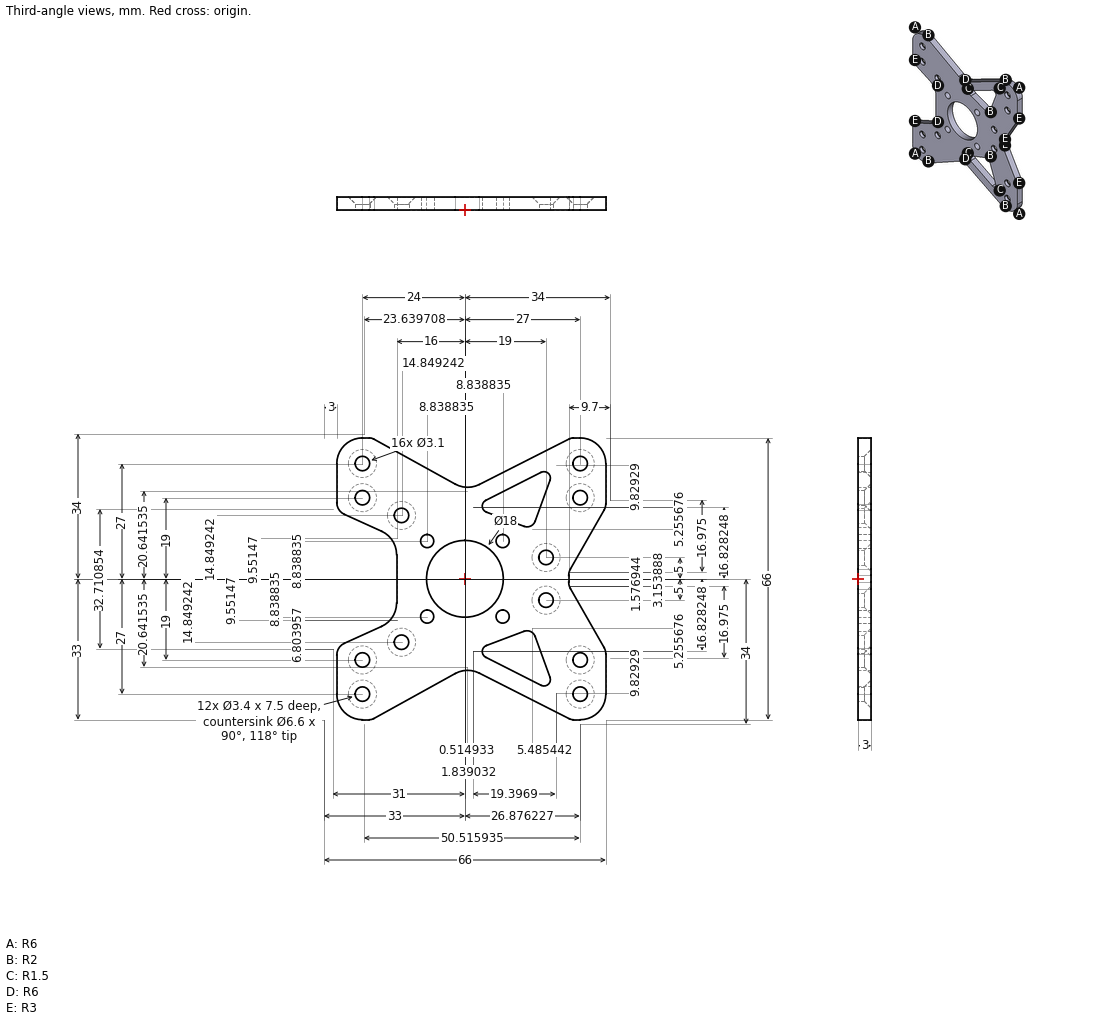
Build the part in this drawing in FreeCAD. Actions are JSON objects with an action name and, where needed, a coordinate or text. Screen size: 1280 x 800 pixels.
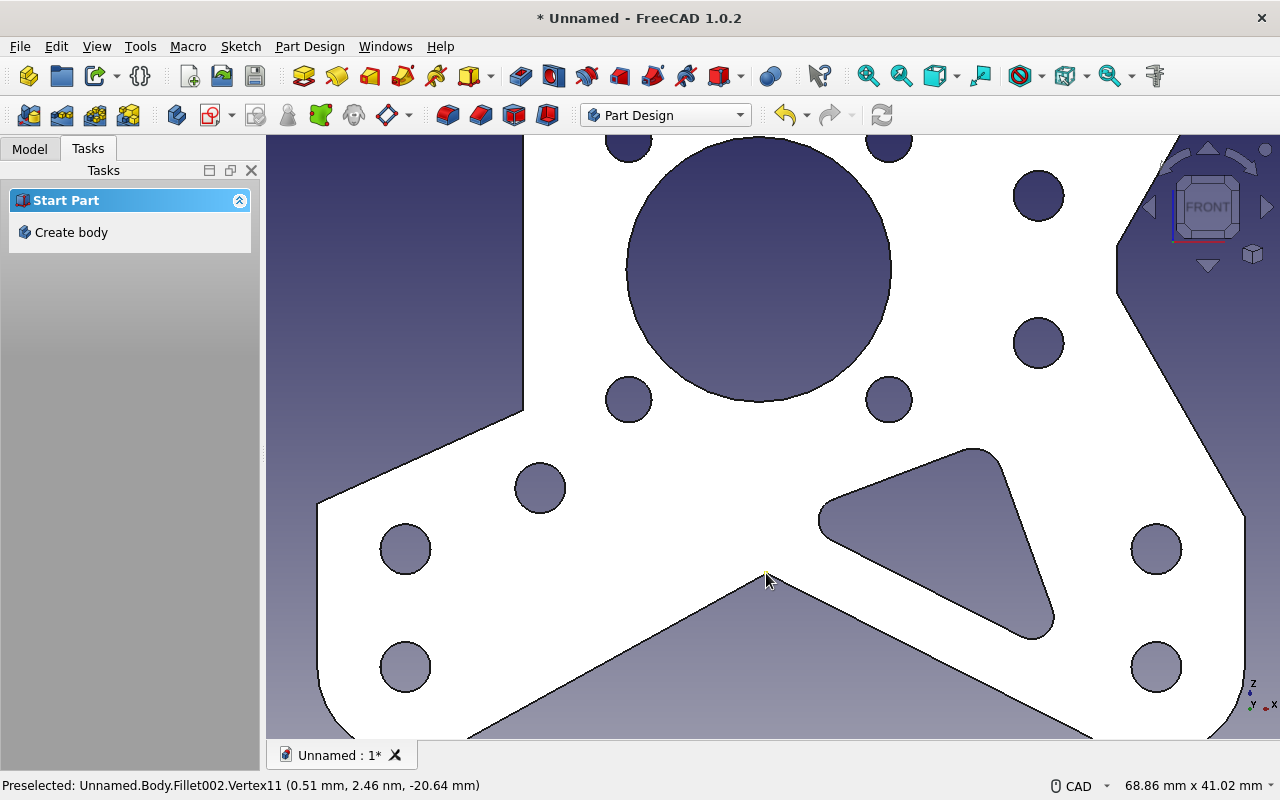
{"action": "left_click", "coordinate": [869, 76]}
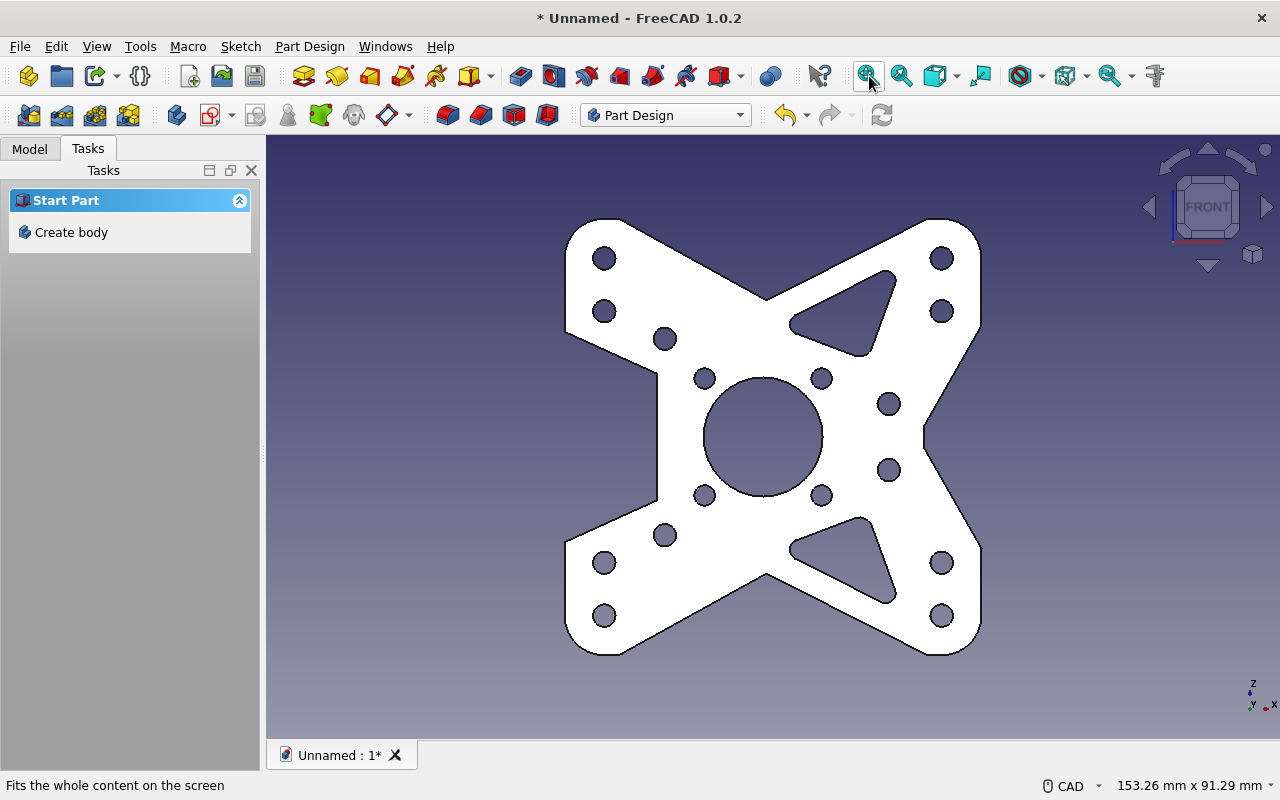
{"action": "key", "text": "3"}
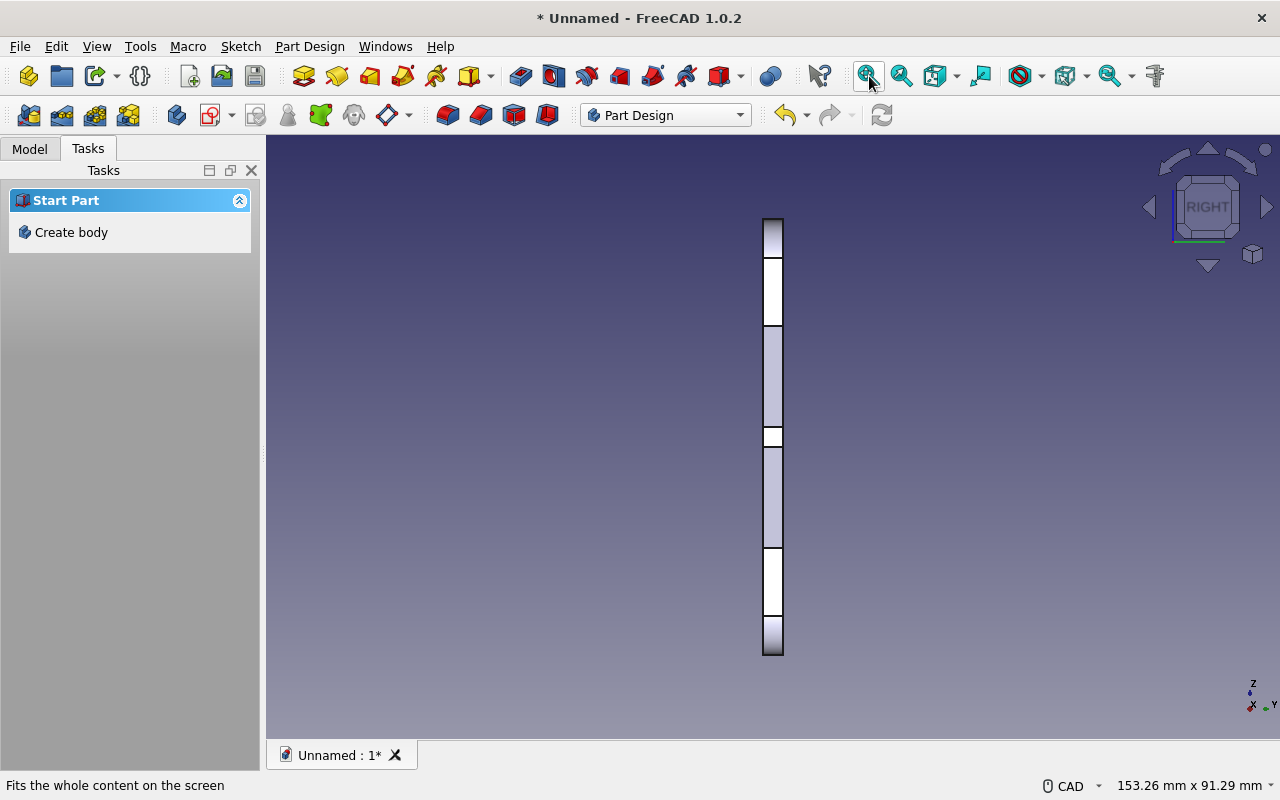
{"action": "scroll", "coordinate": [773, 573], "scroll_direction": "up", "scroll_amount": 4}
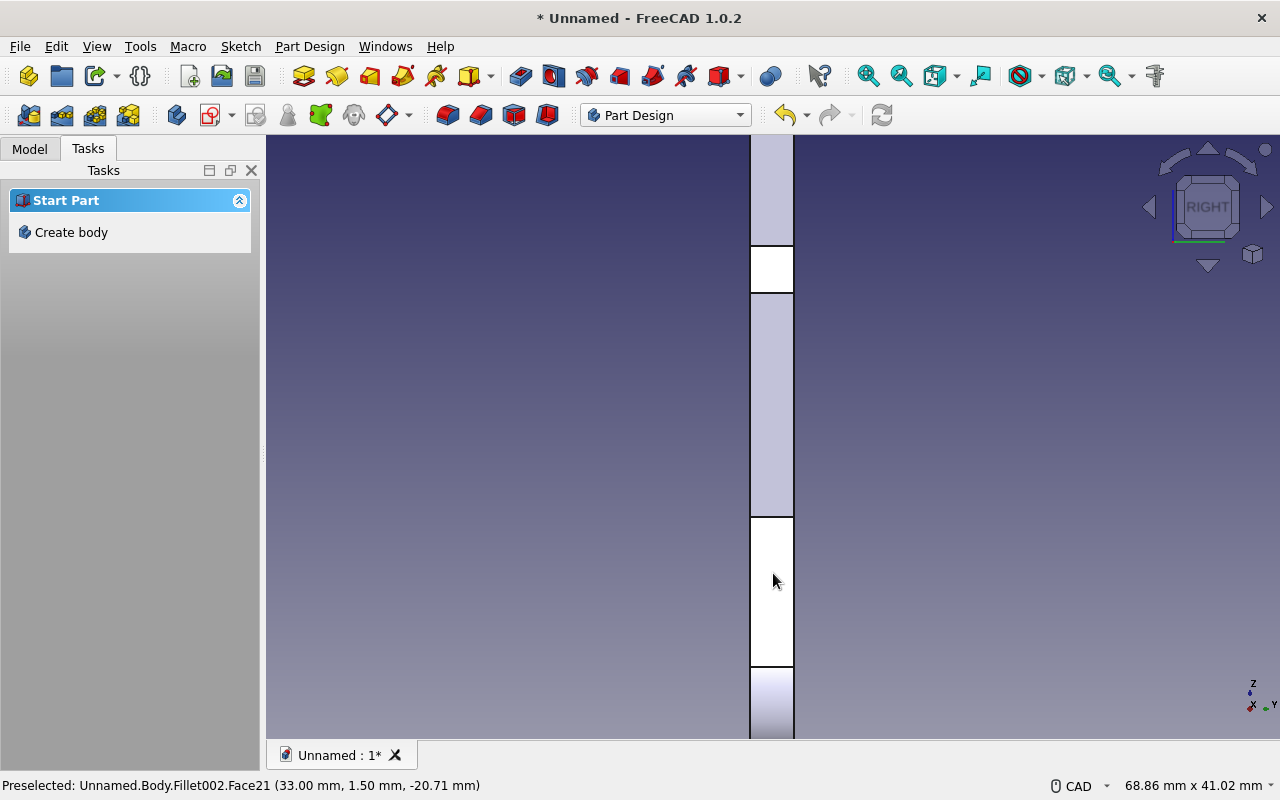
{"action": "left_click", "coordinate": [869, 76]}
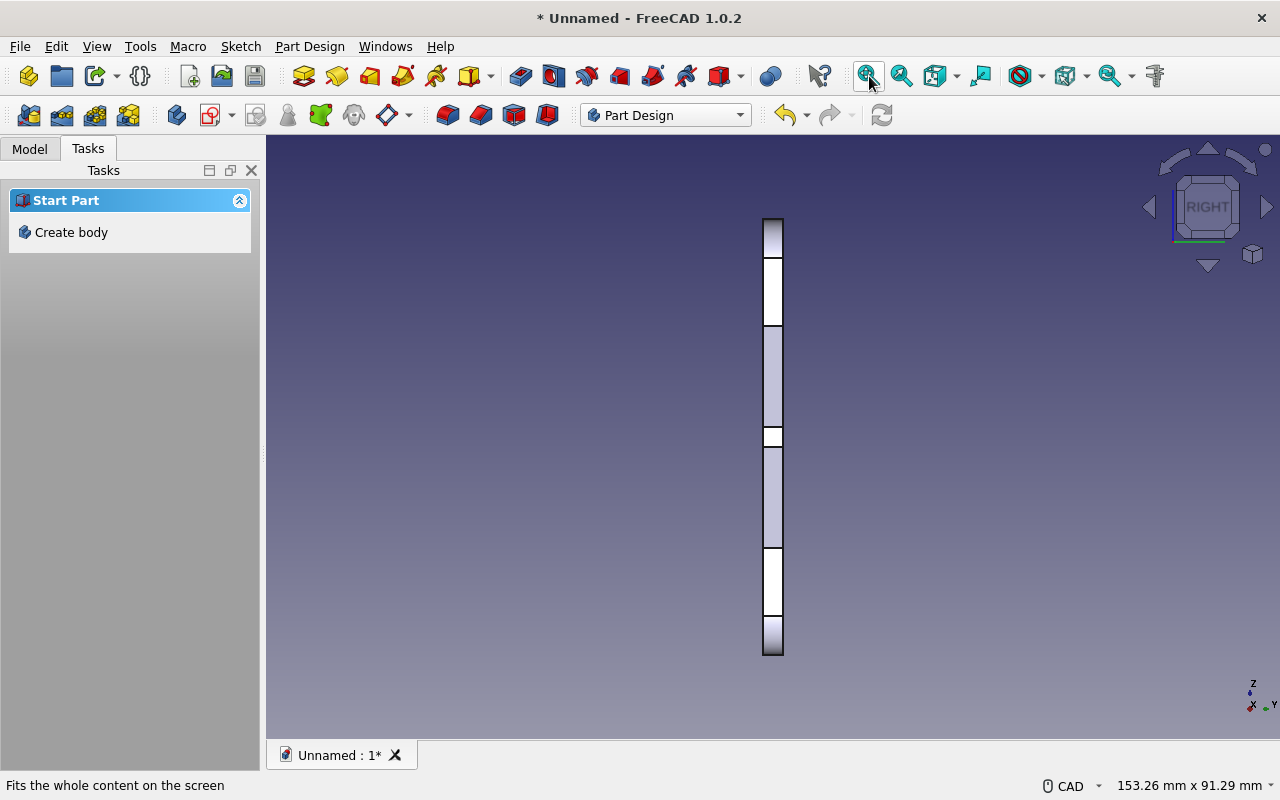
{"action": "key", "text": "5"}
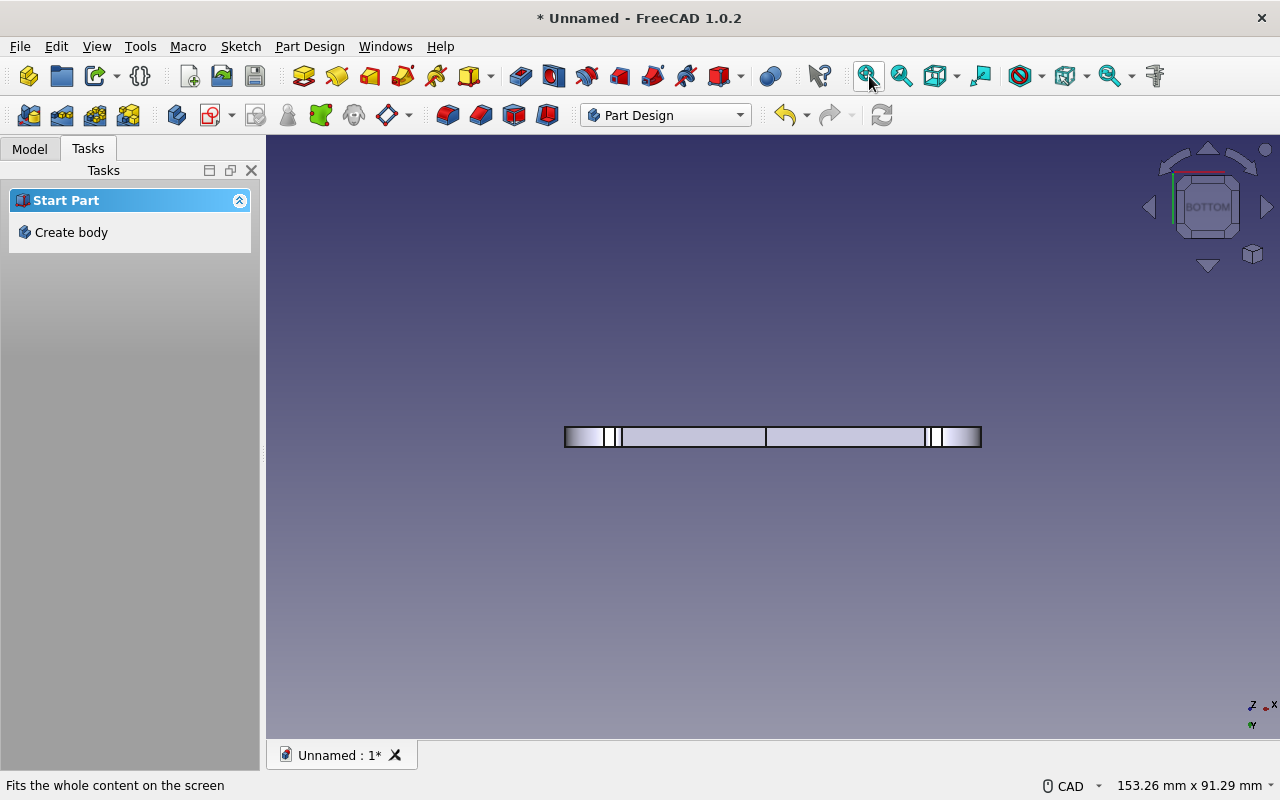
{"action": "left_click", "coordinate": [869, 76]}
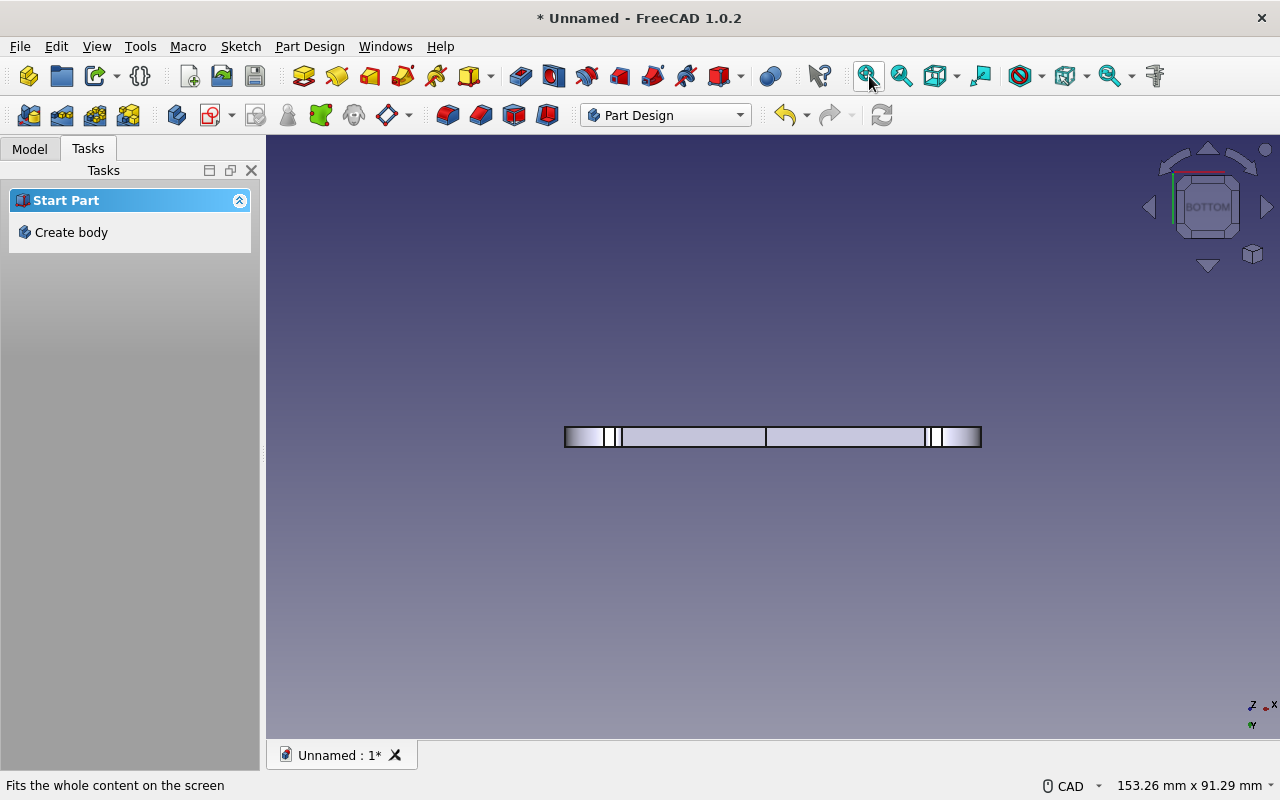
{"action": "scroll", "coordinate": [766, 436], "scroll_direction": "up", "scroll_amount": 4}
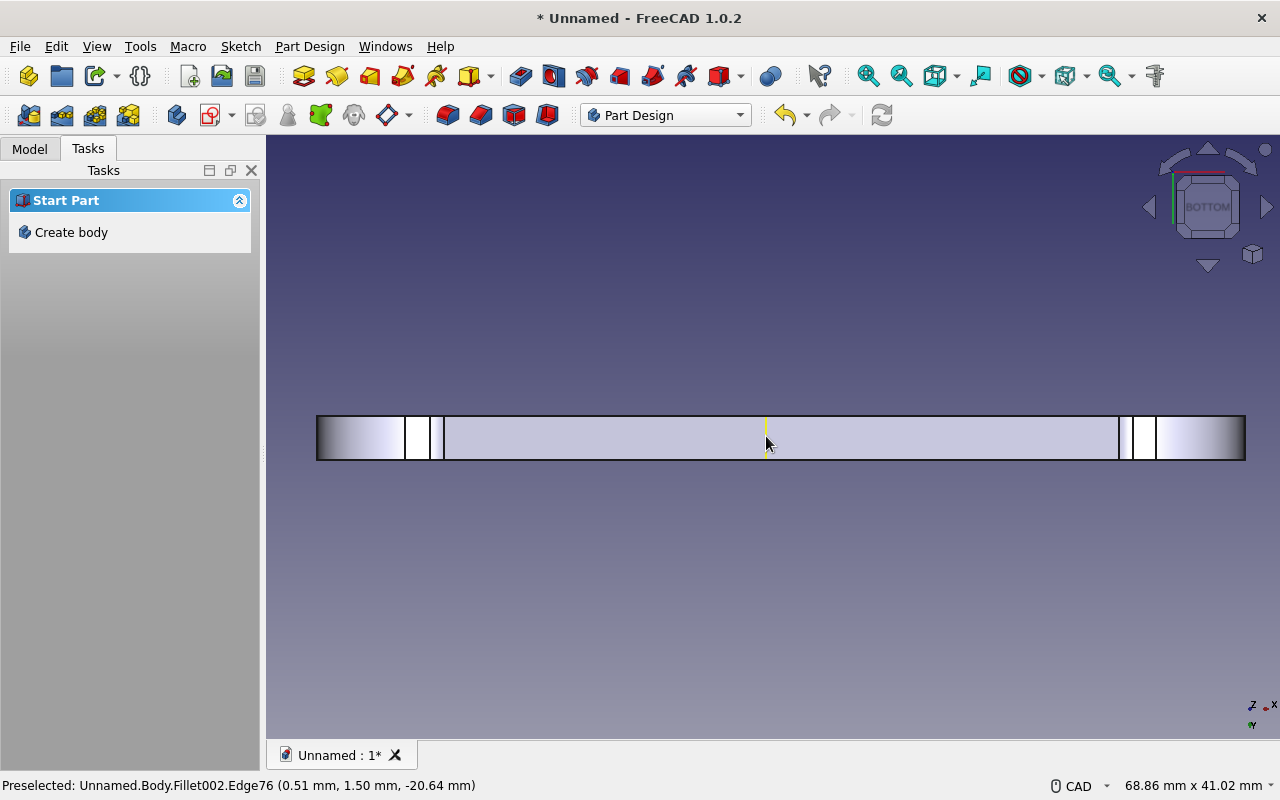
{"action": "left_click", "coordinate": [869, 76]}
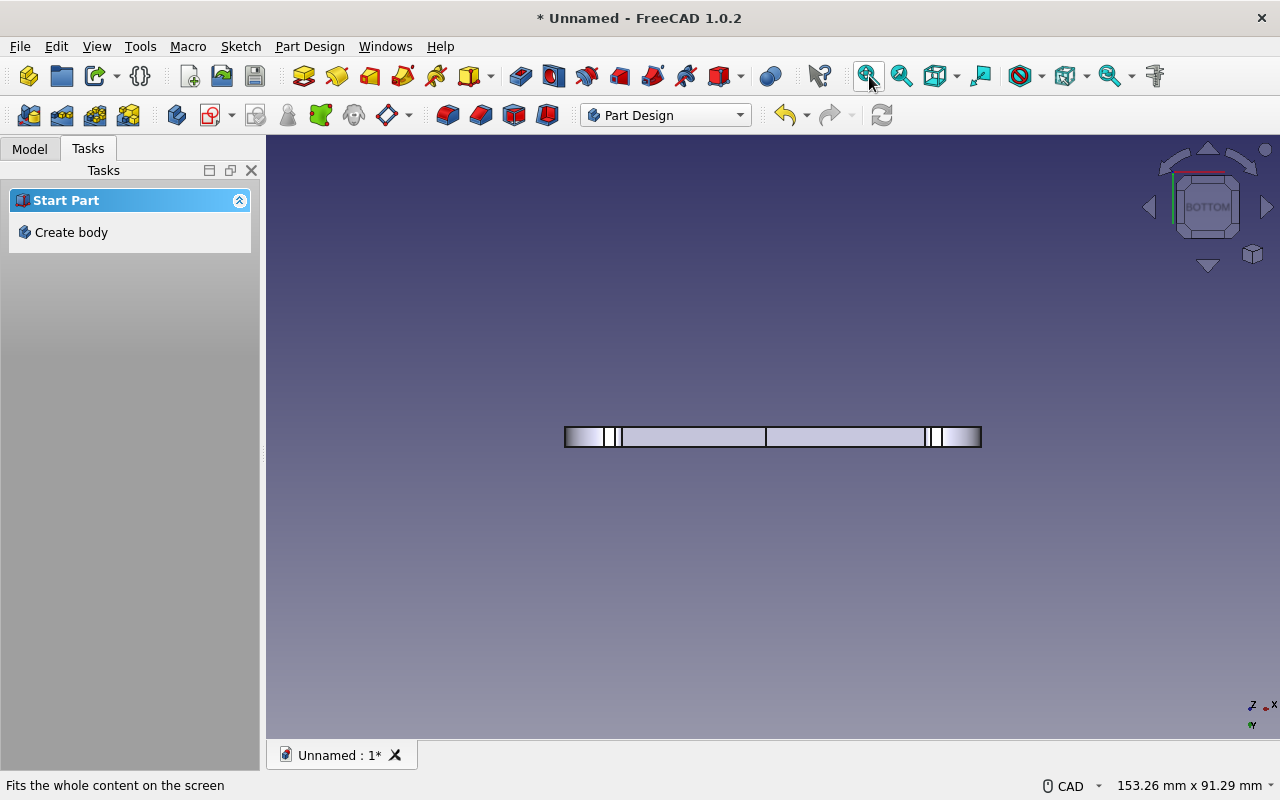
{"action": "key", "text": "4"}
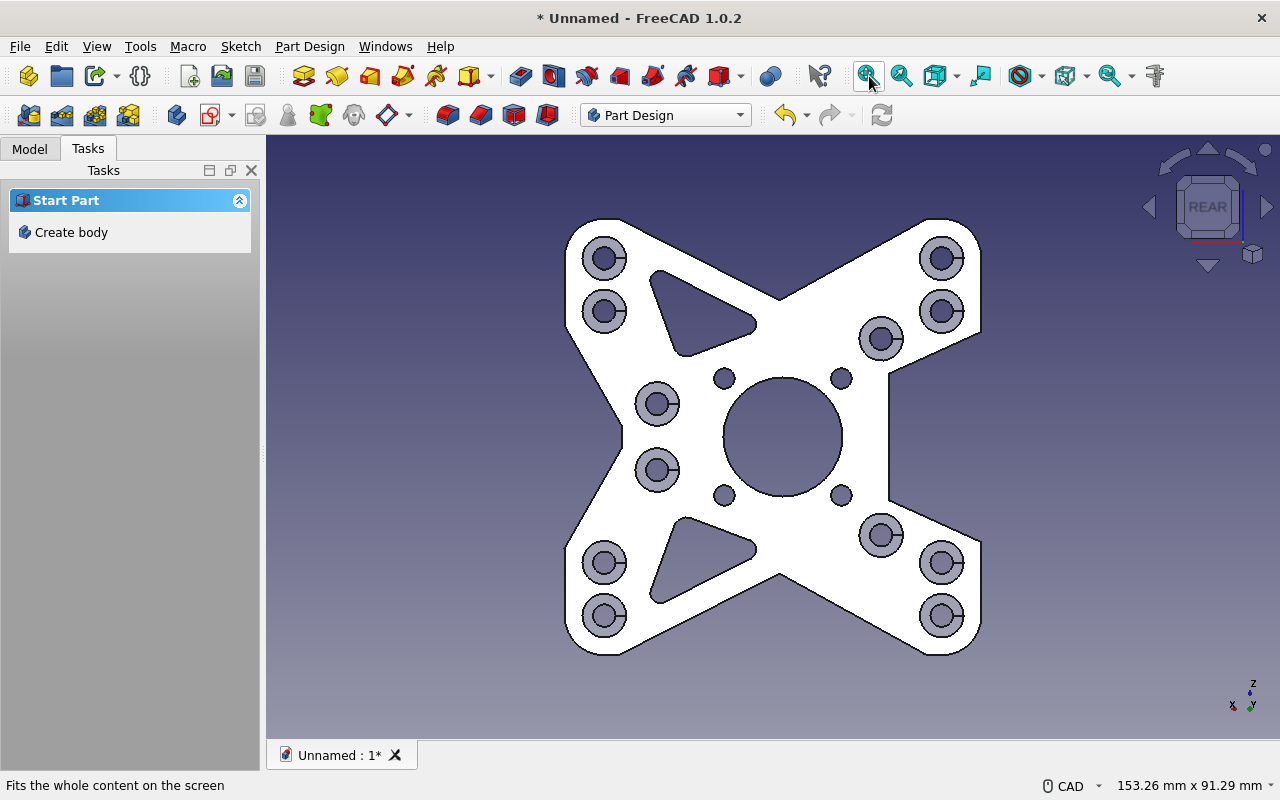
{"action": "scroll", "coordinate": [780, 573], "scroll_direction": "up", "scroll_amount": 4}